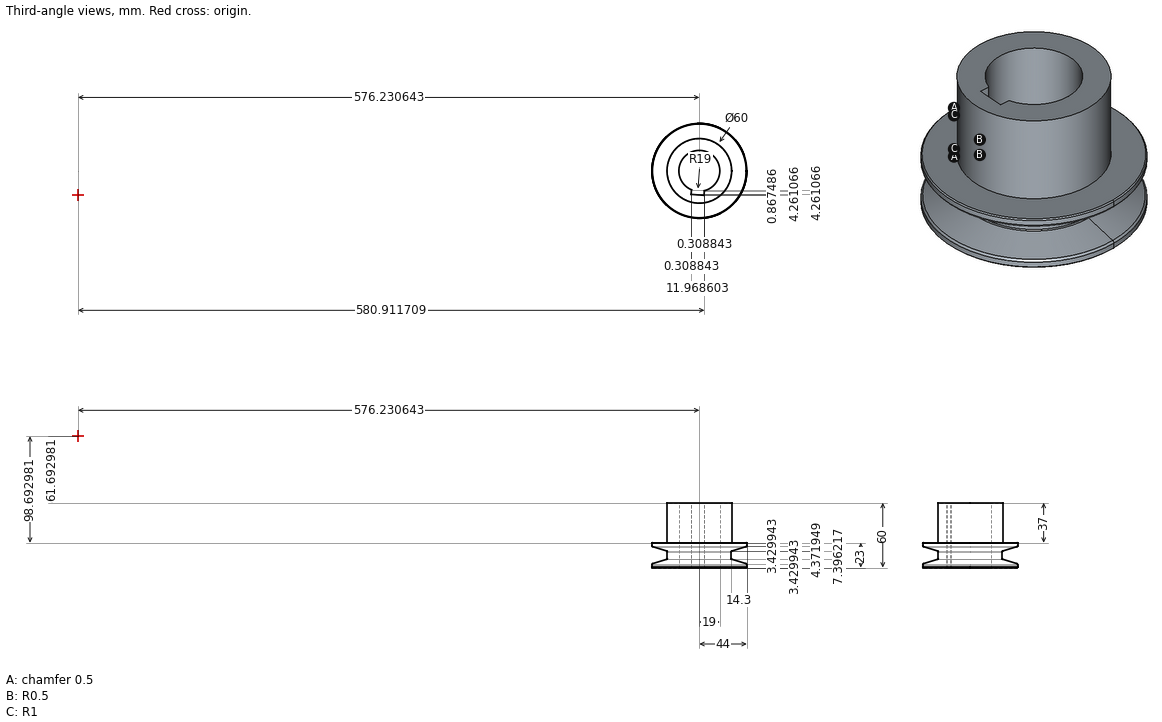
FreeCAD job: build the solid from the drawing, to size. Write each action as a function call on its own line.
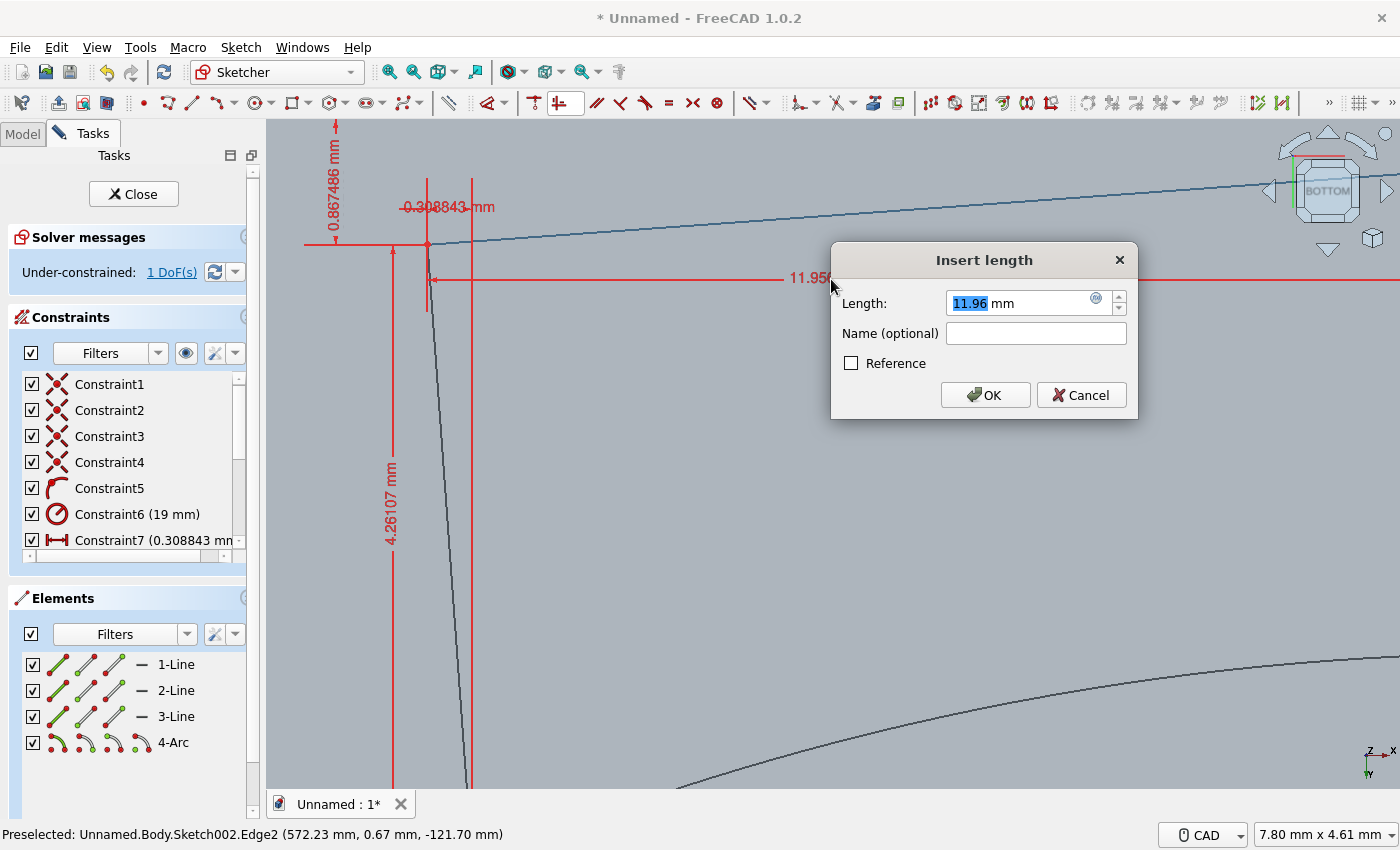
text(11.968603)
key(Return)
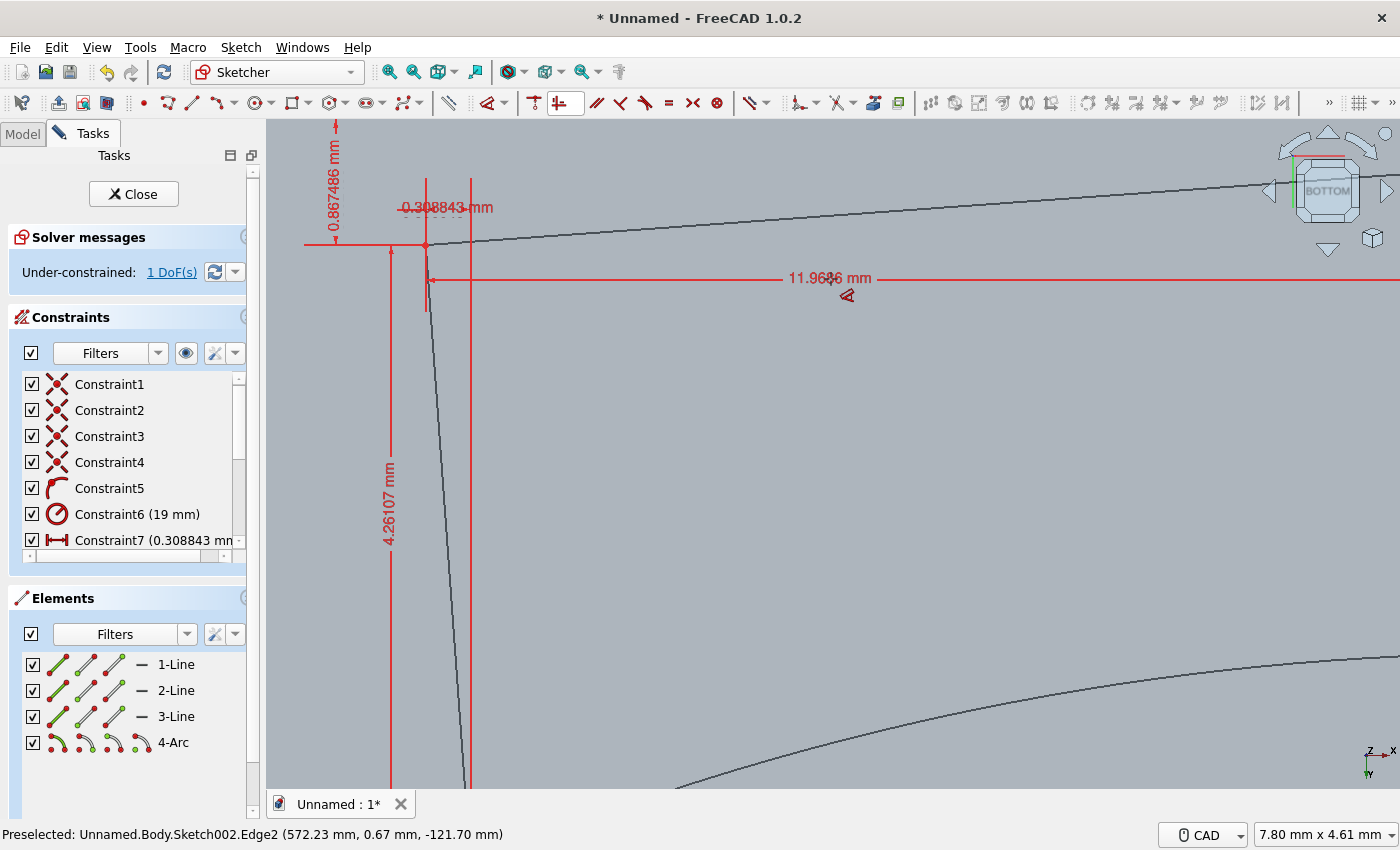
scroll(442, 432, down, 5)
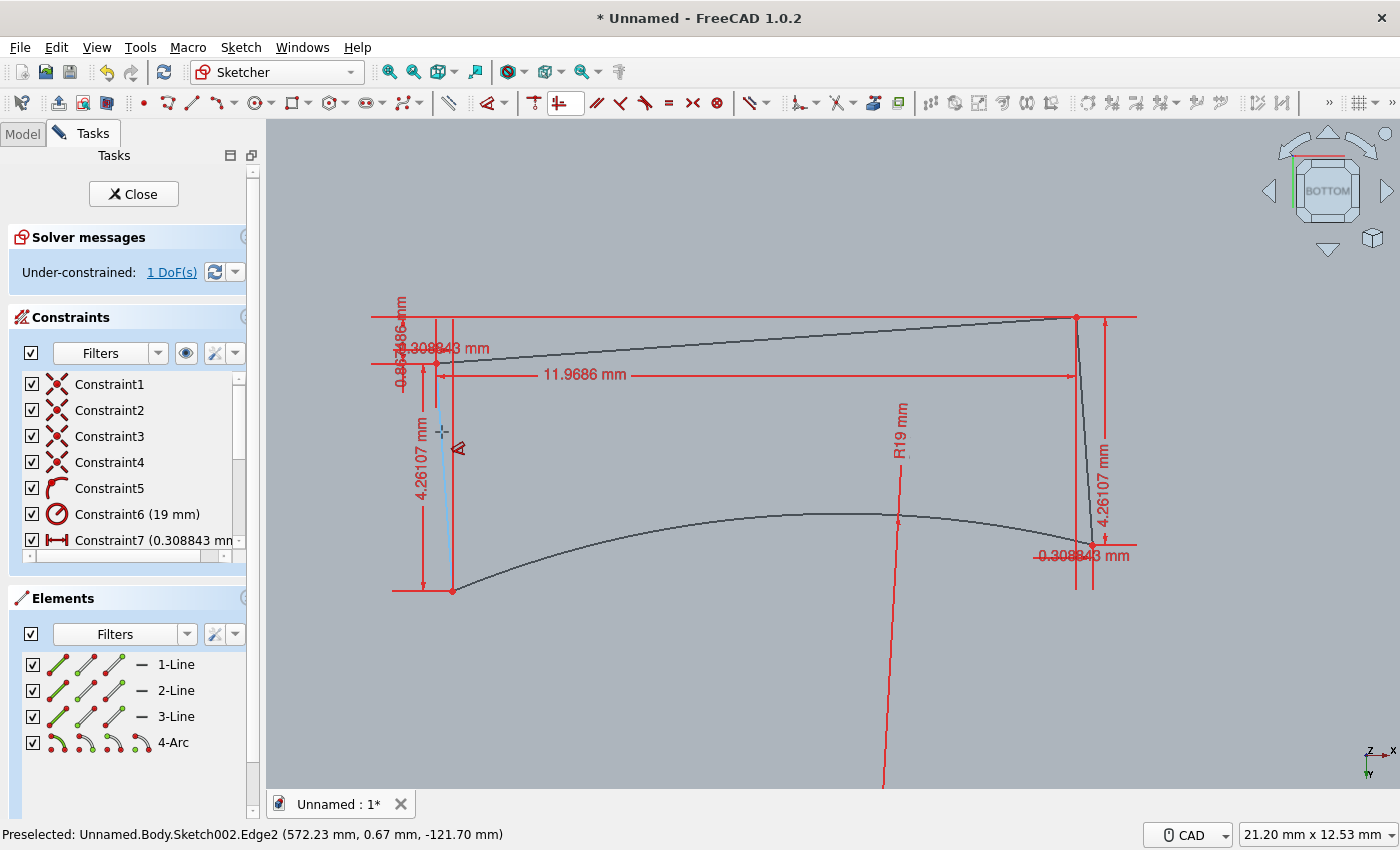
click(1093, 545)
click(693, 511)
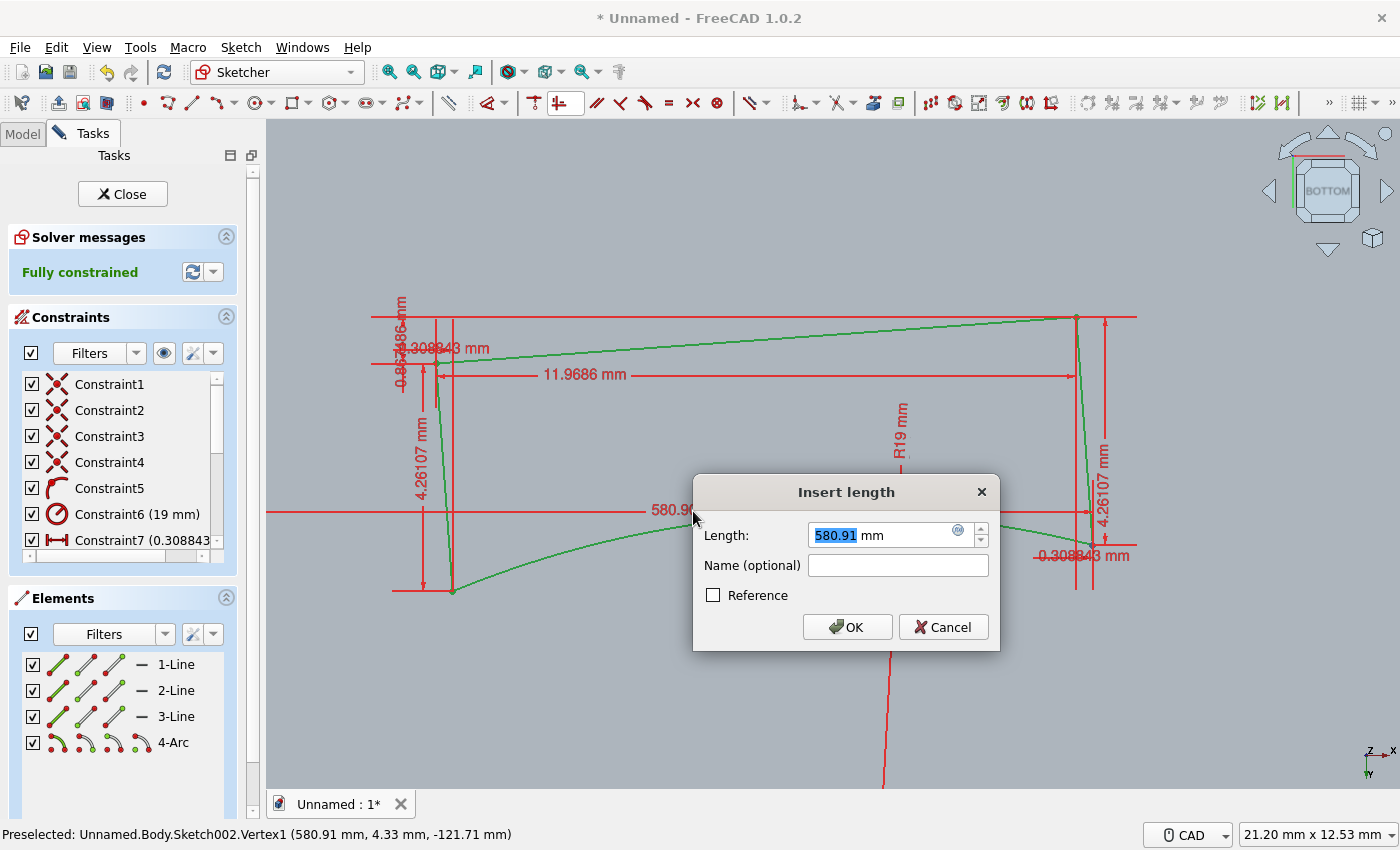
text(580.911709)
key(Return)
key(Escape)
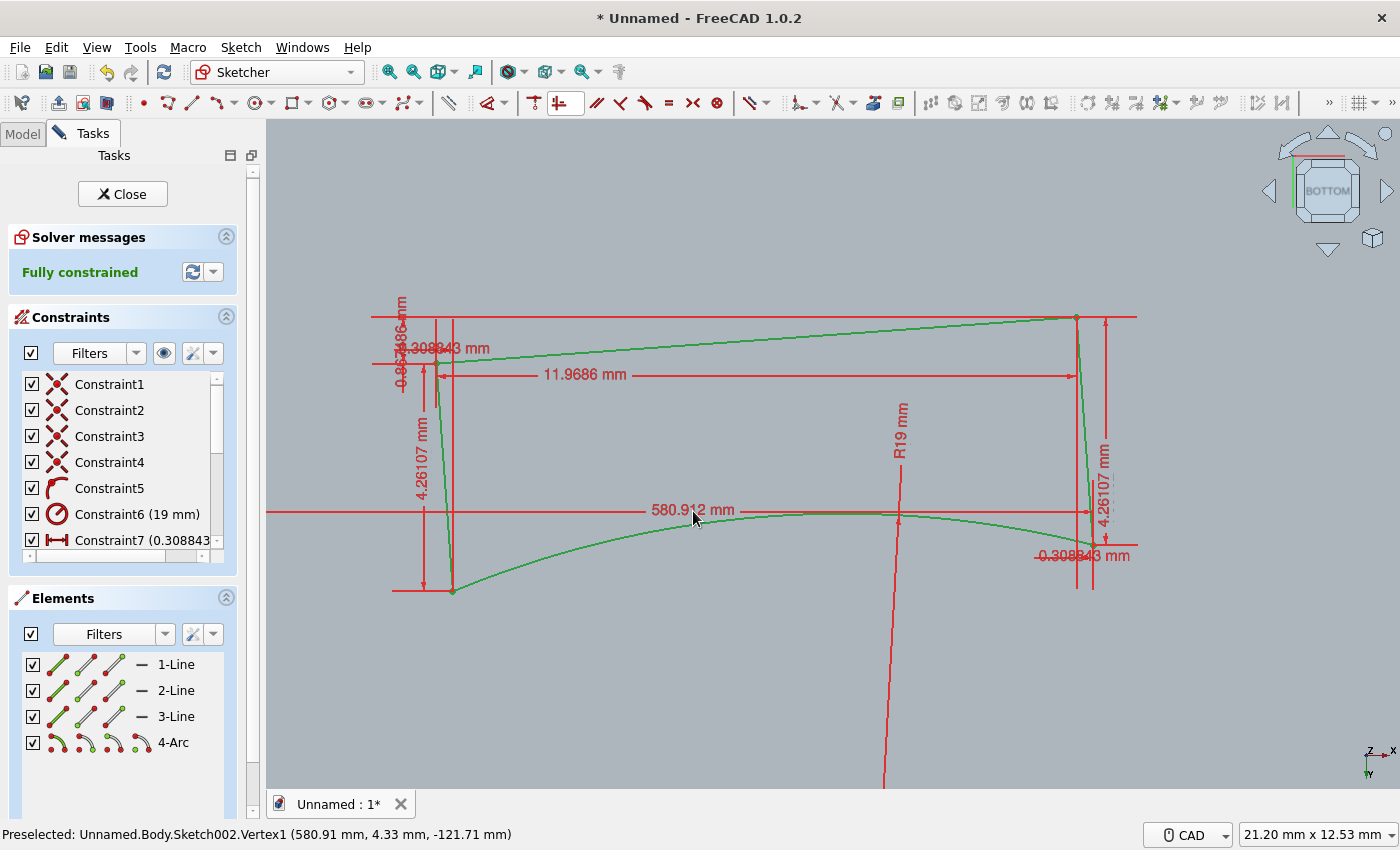
click(123, 194)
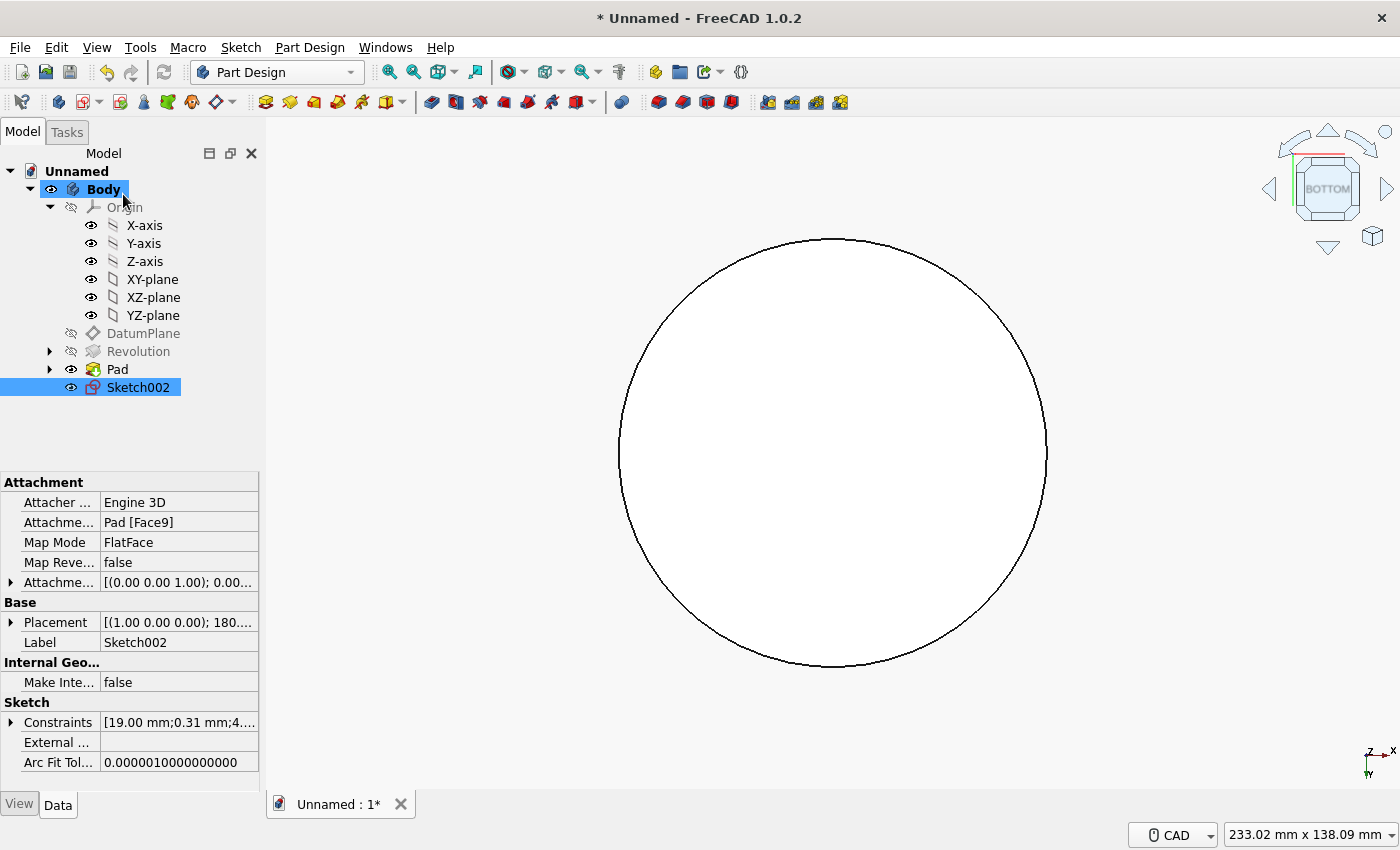
click(432, 102)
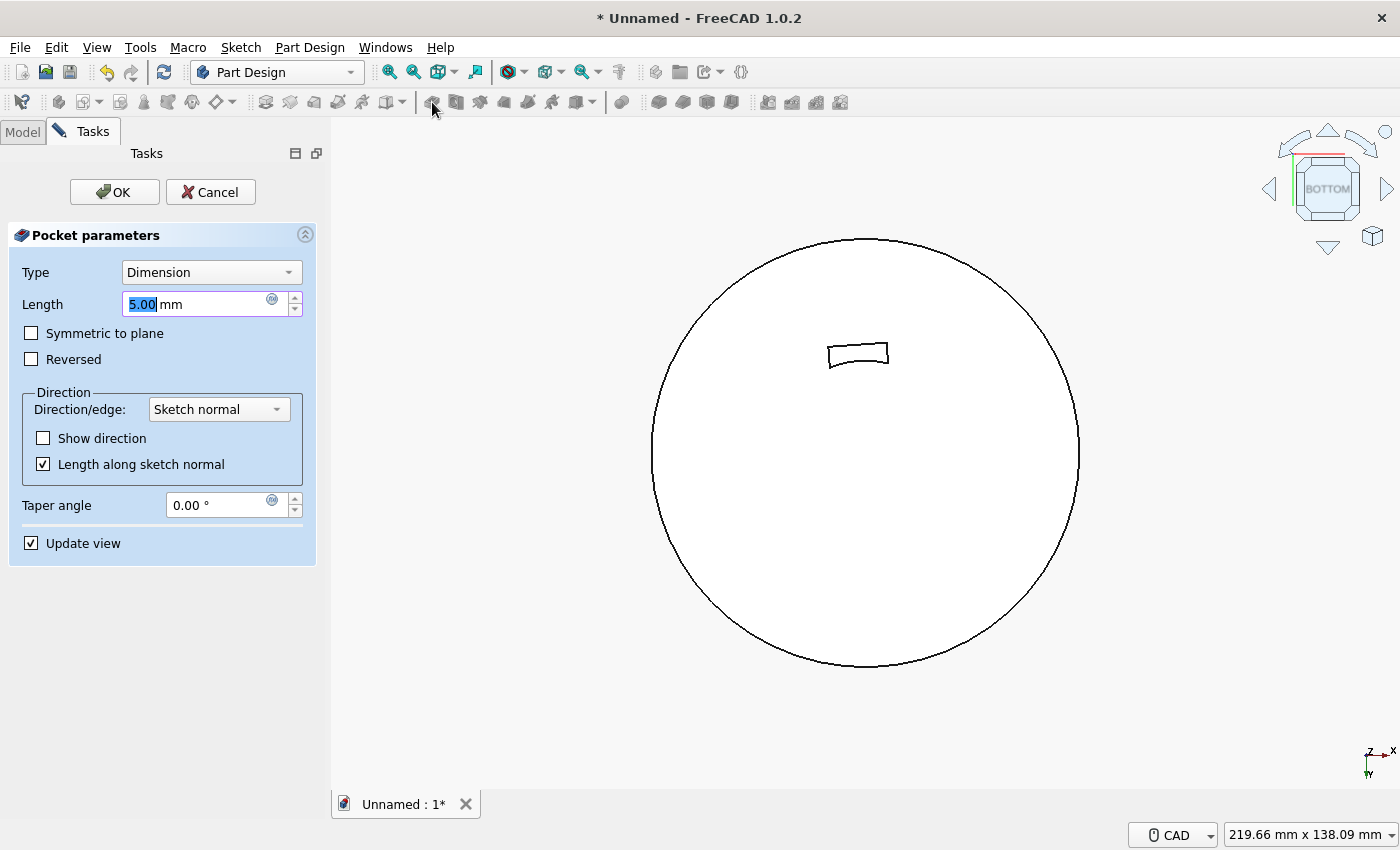
click(212, 272)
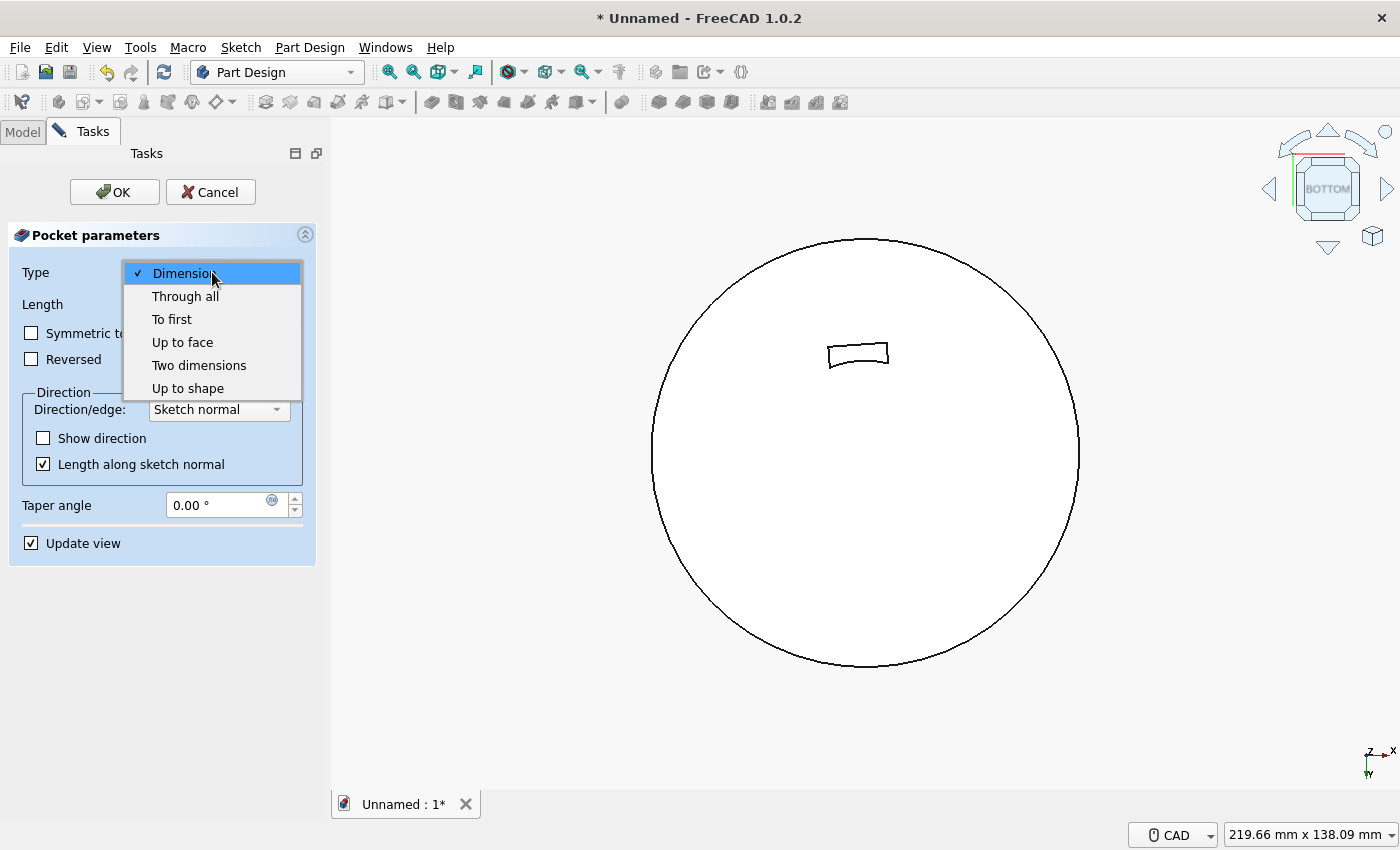
click(212, 296)